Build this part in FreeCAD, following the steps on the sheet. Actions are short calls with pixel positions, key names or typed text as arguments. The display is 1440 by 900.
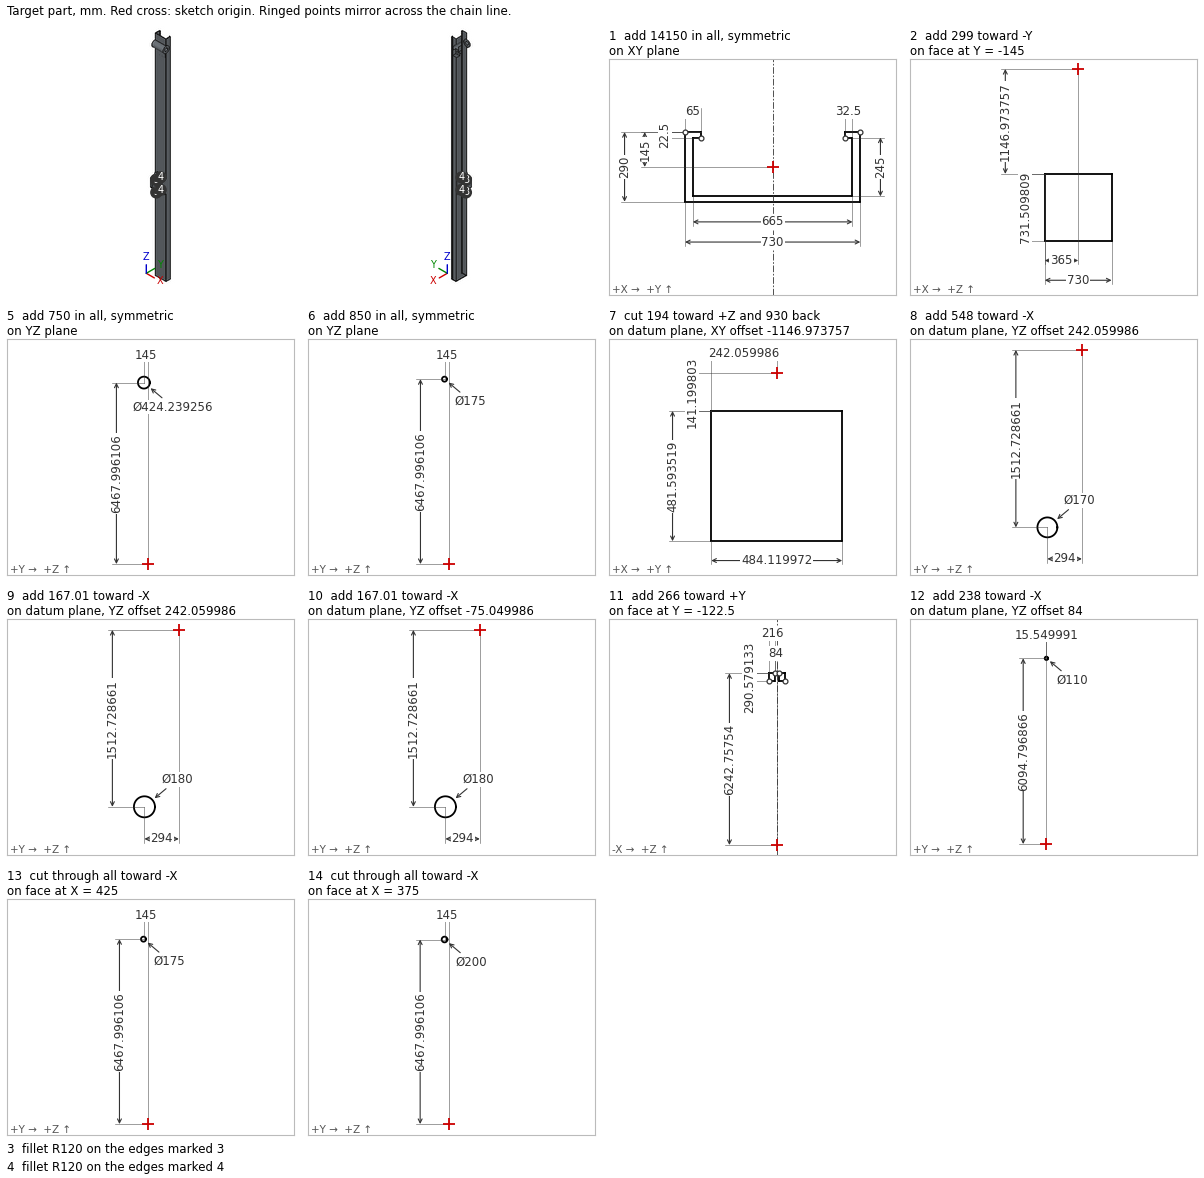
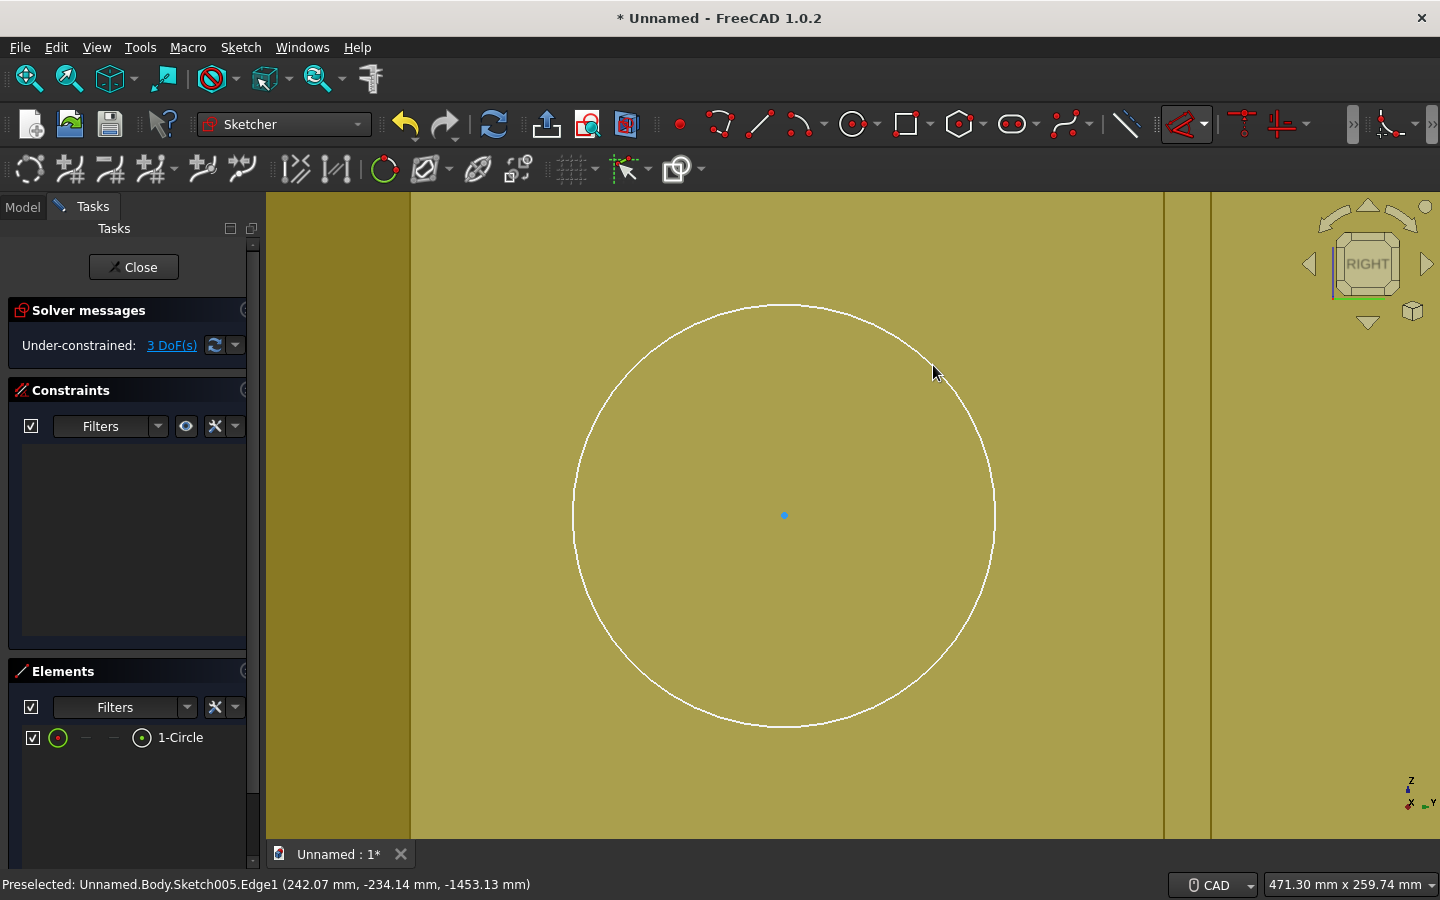
click(933, 366)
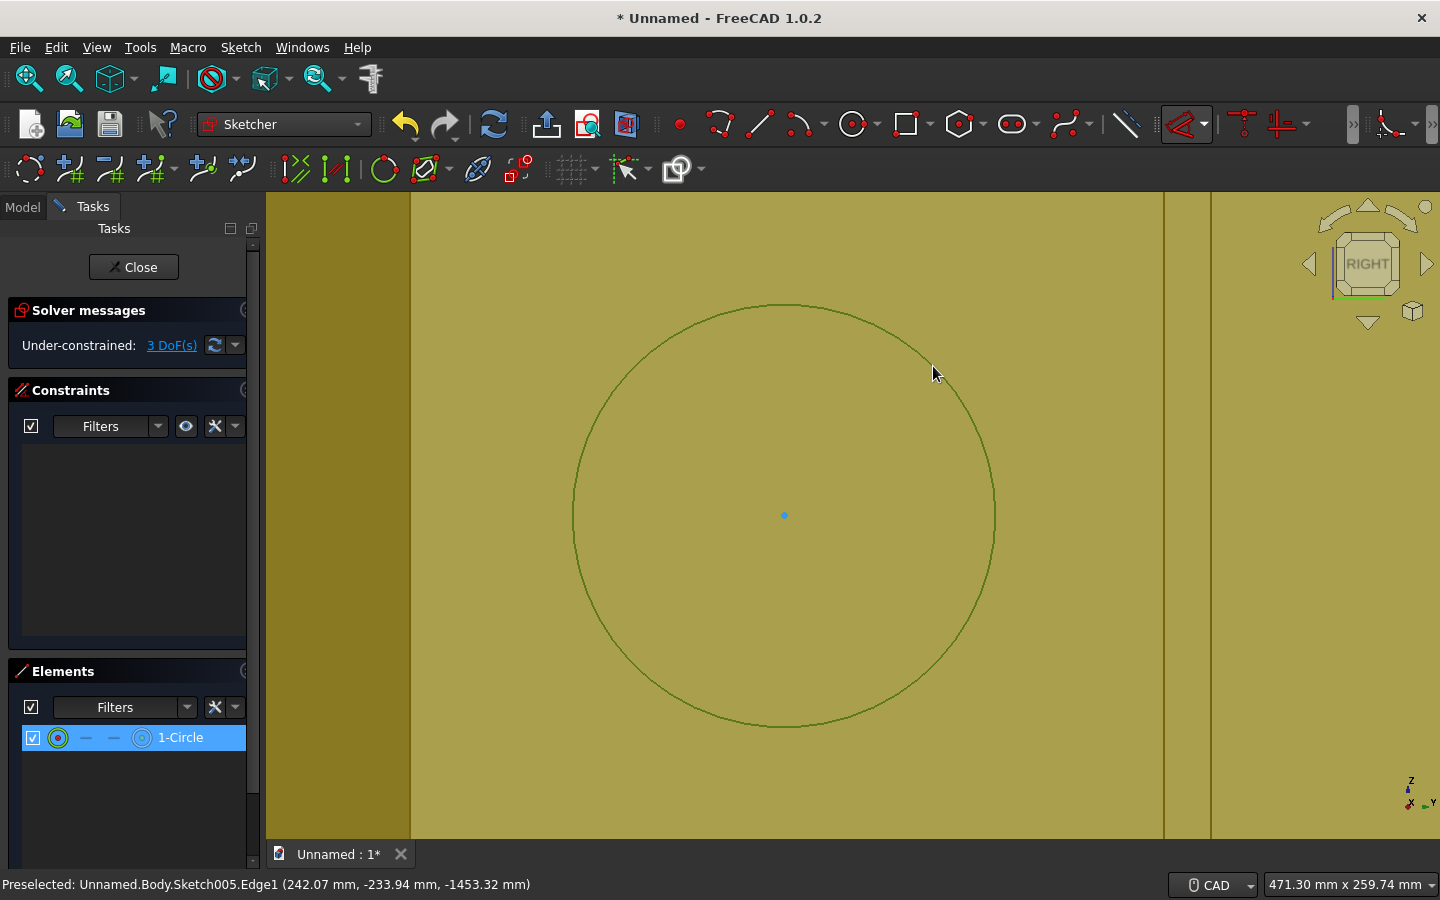
click(1206, 124)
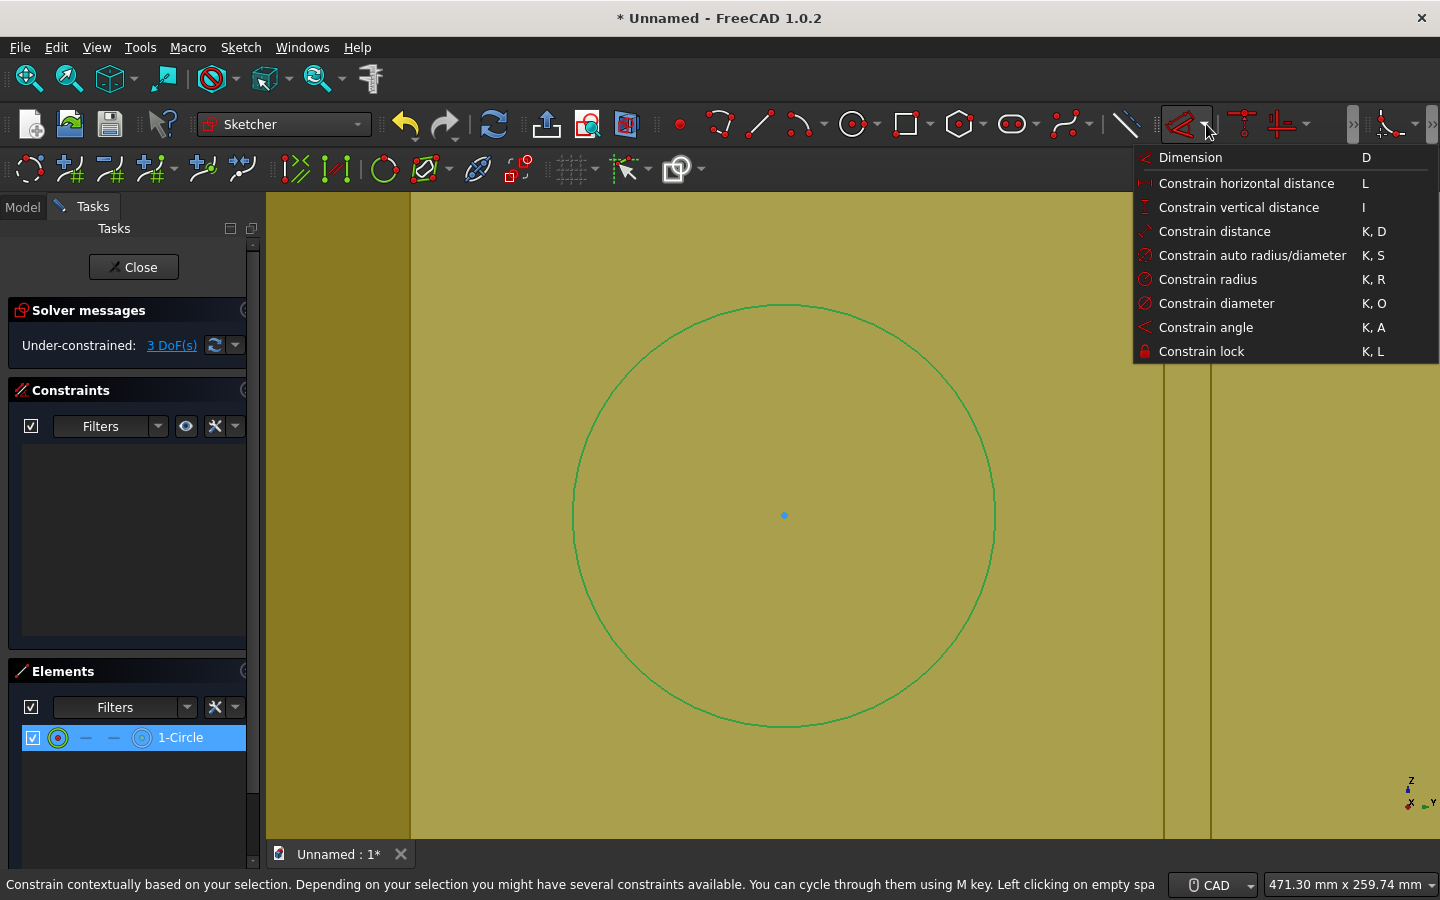
click(1286, 303)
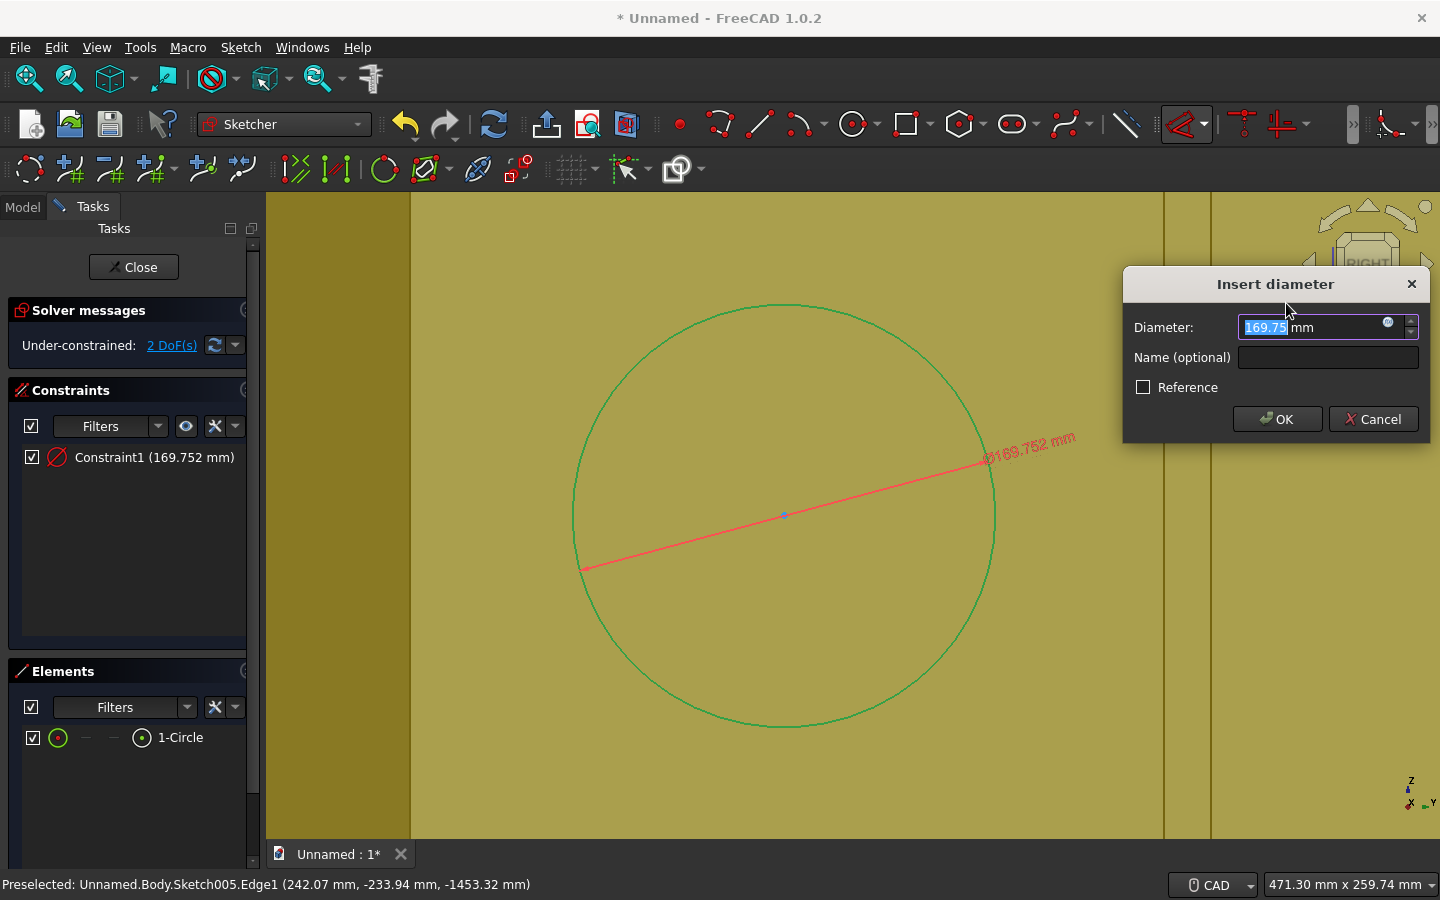
text(170)
key(Return)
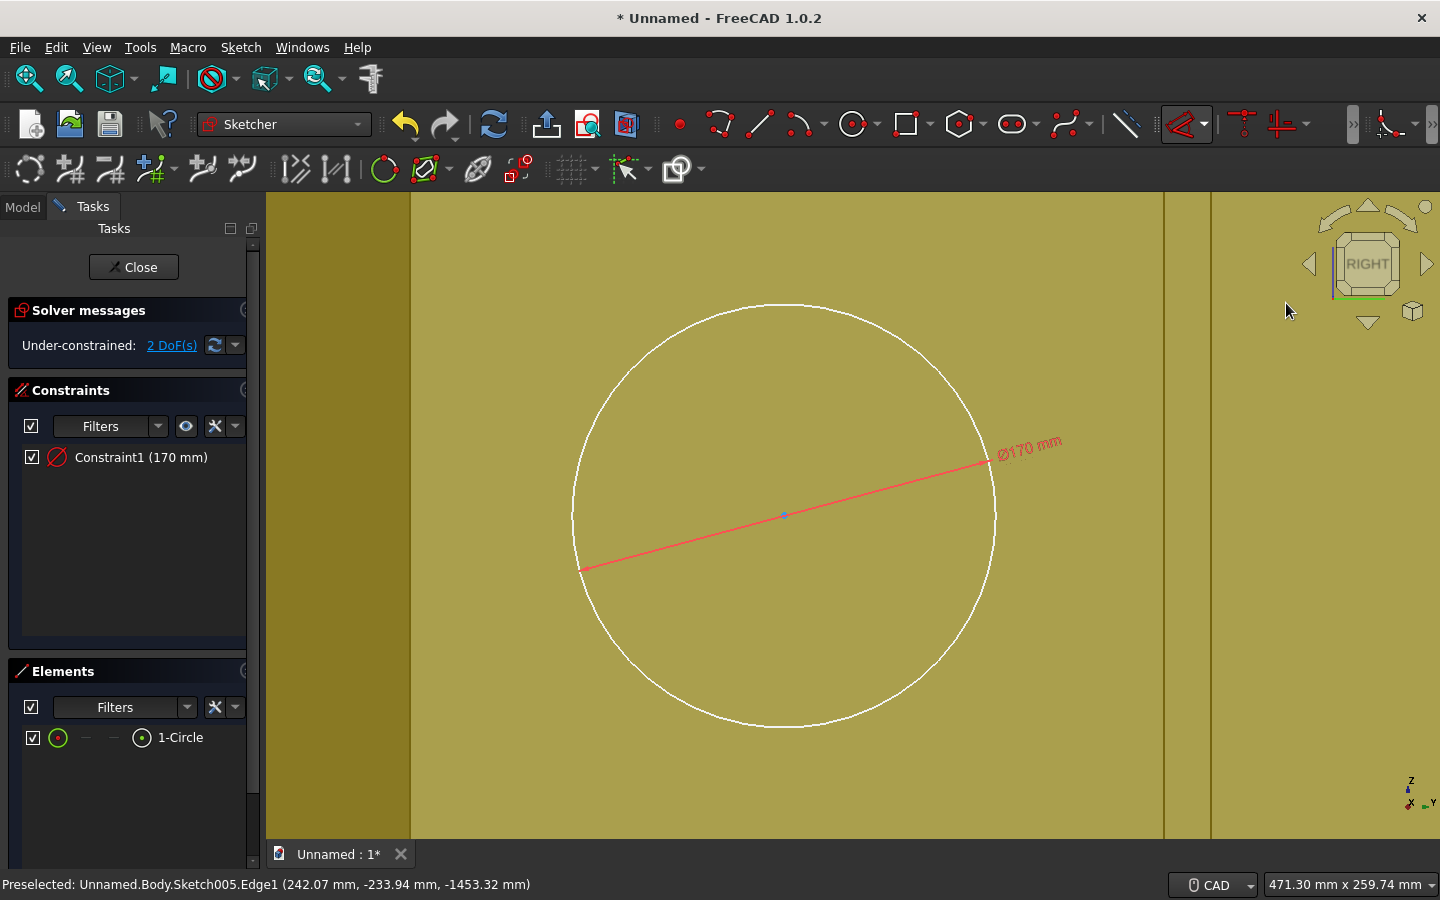
click(784, 516)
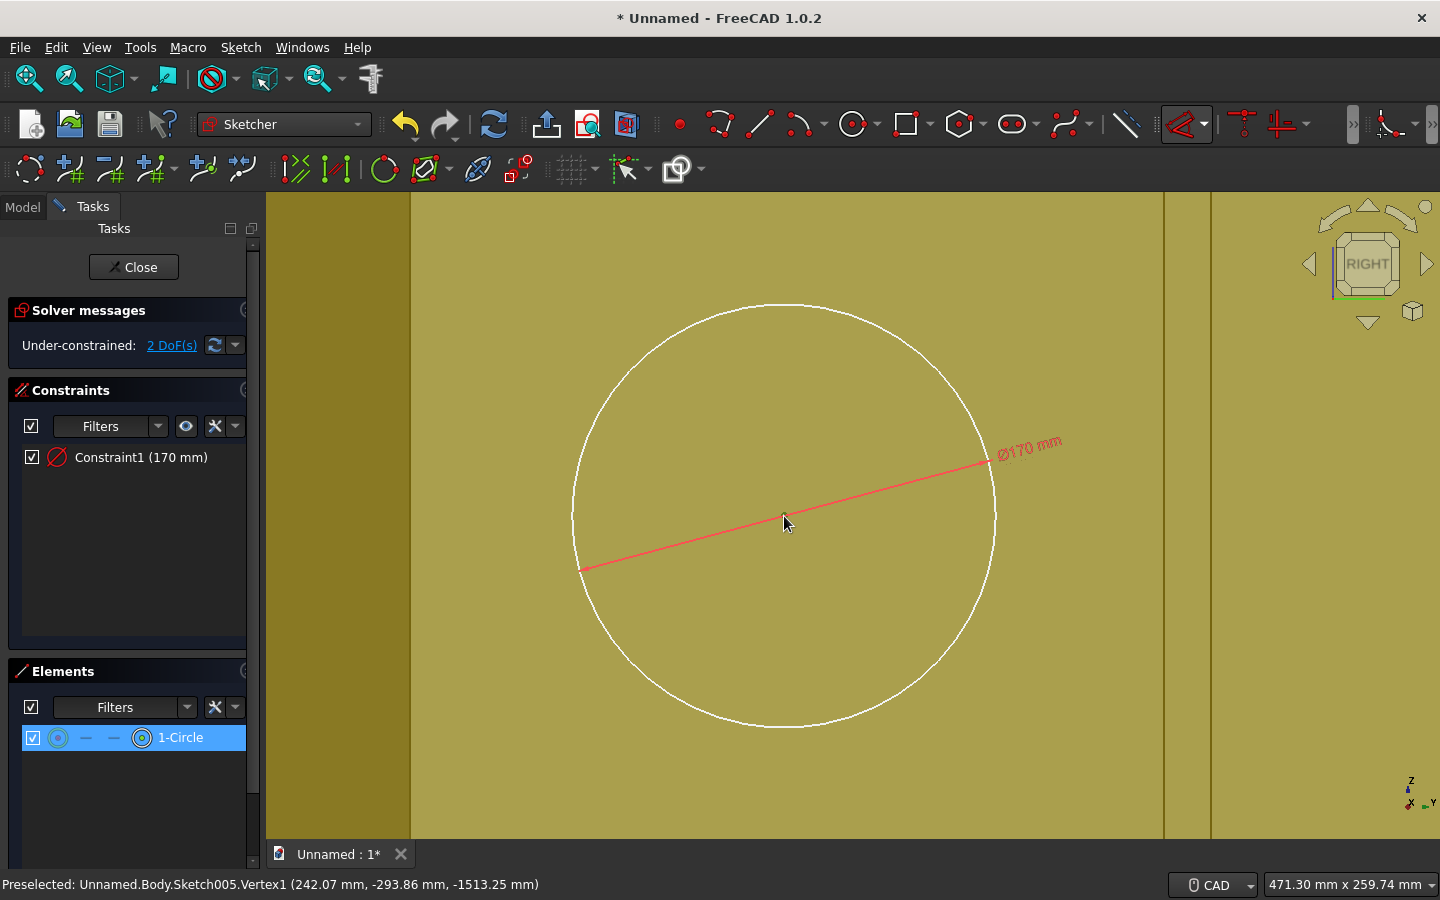
click(1206, 124)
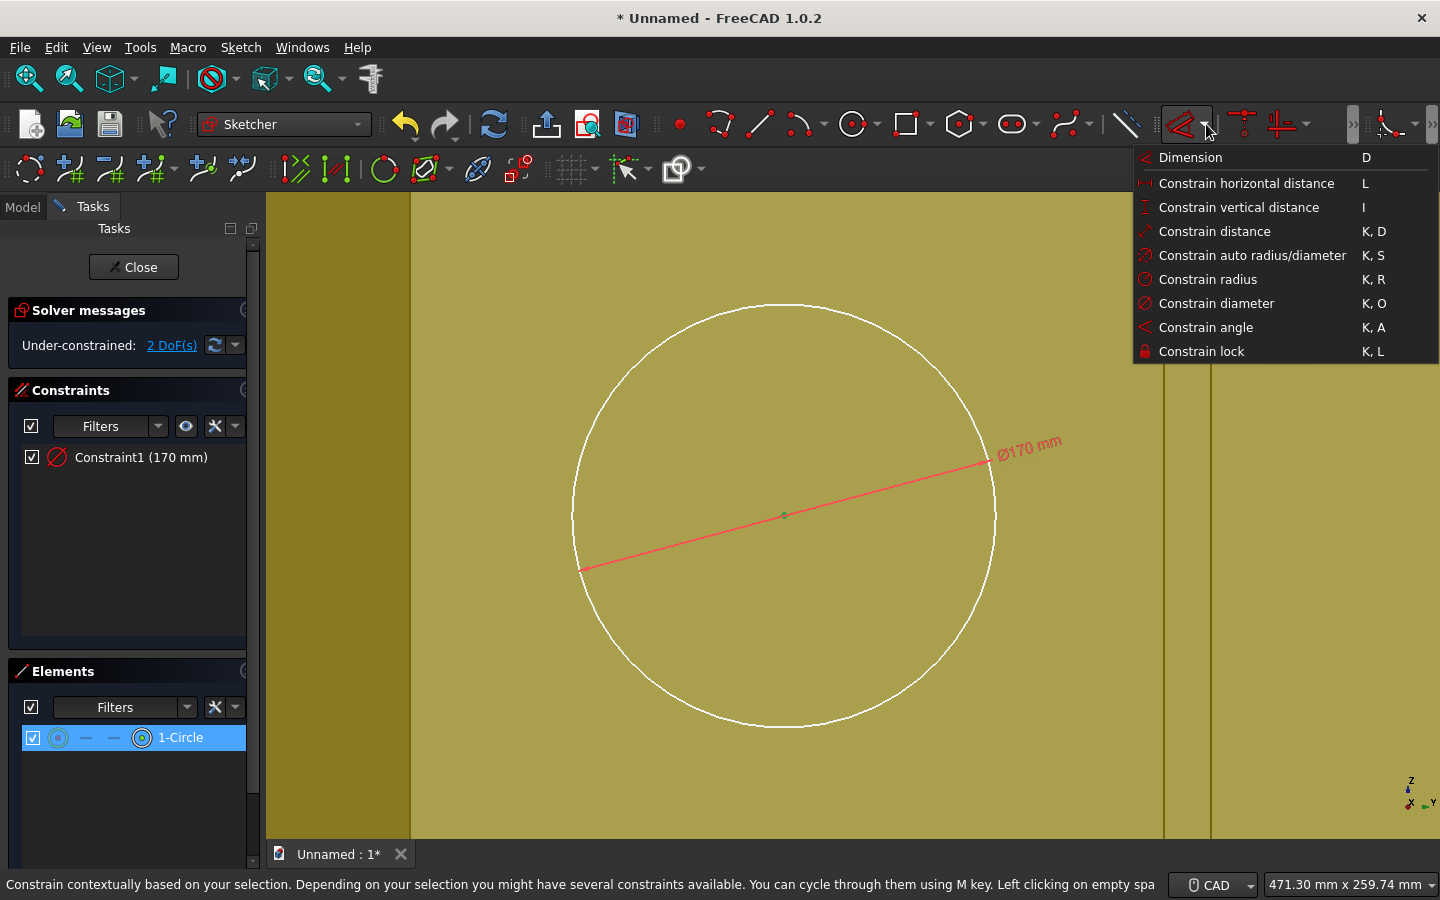
click(1286, 183)